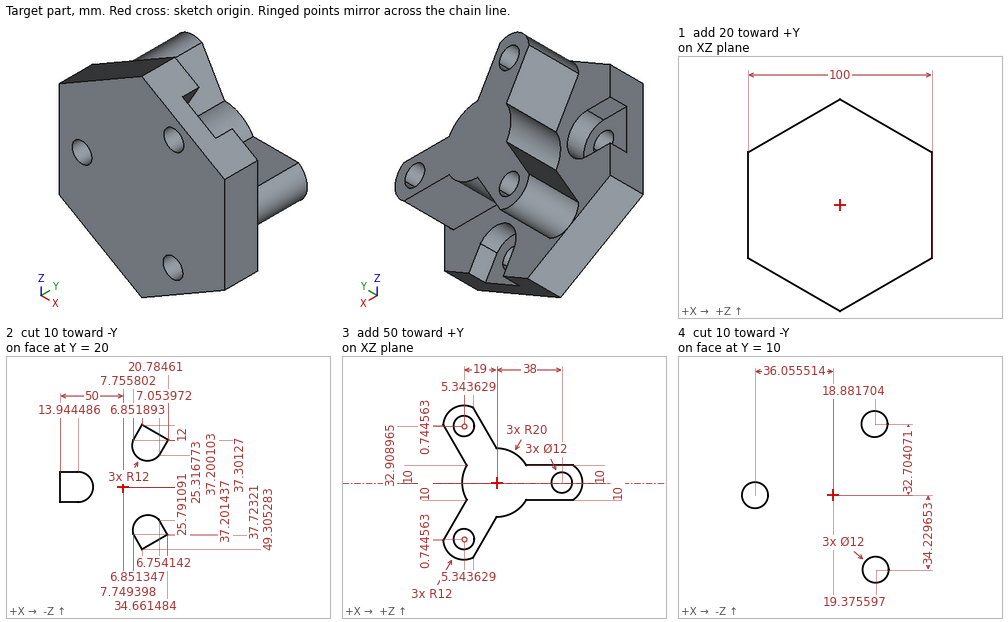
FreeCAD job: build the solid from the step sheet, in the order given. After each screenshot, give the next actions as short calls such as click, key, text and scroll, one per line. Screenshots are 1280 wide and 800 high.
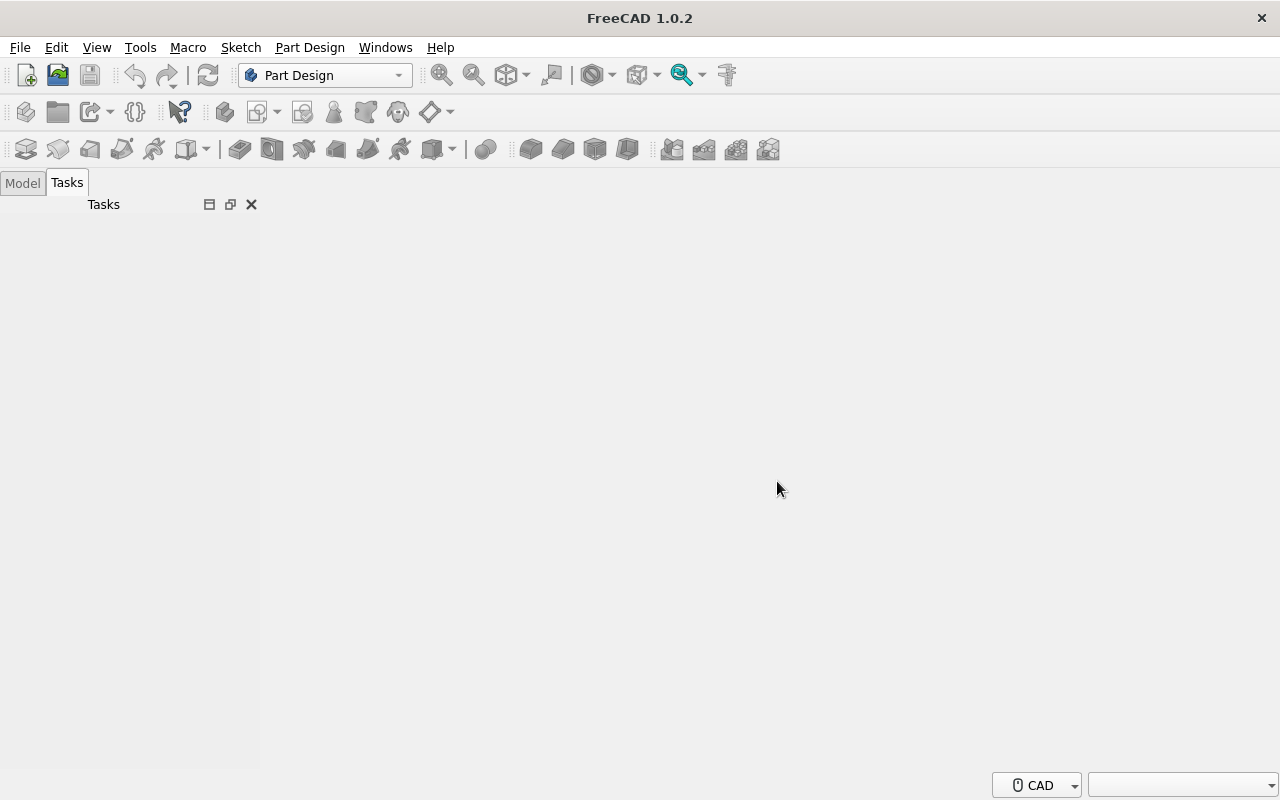
click(26, 76)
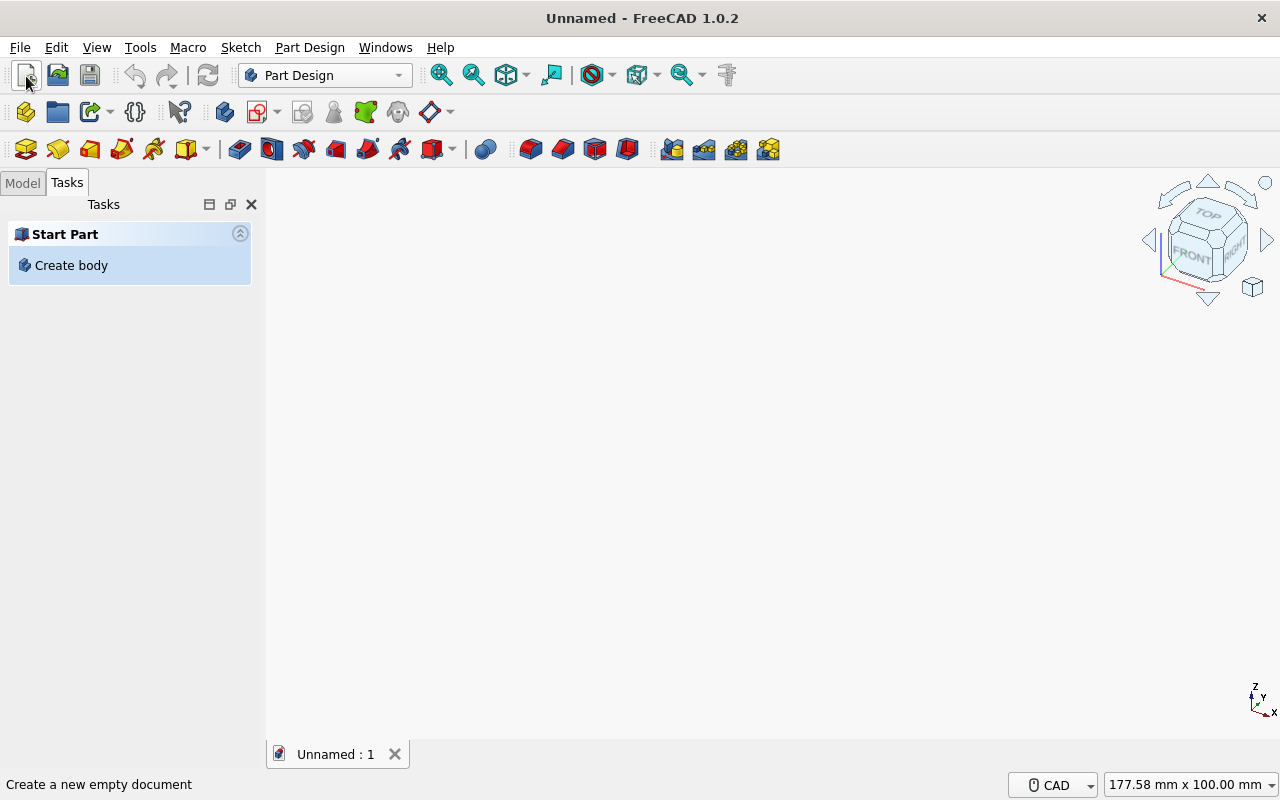
click(258, 112)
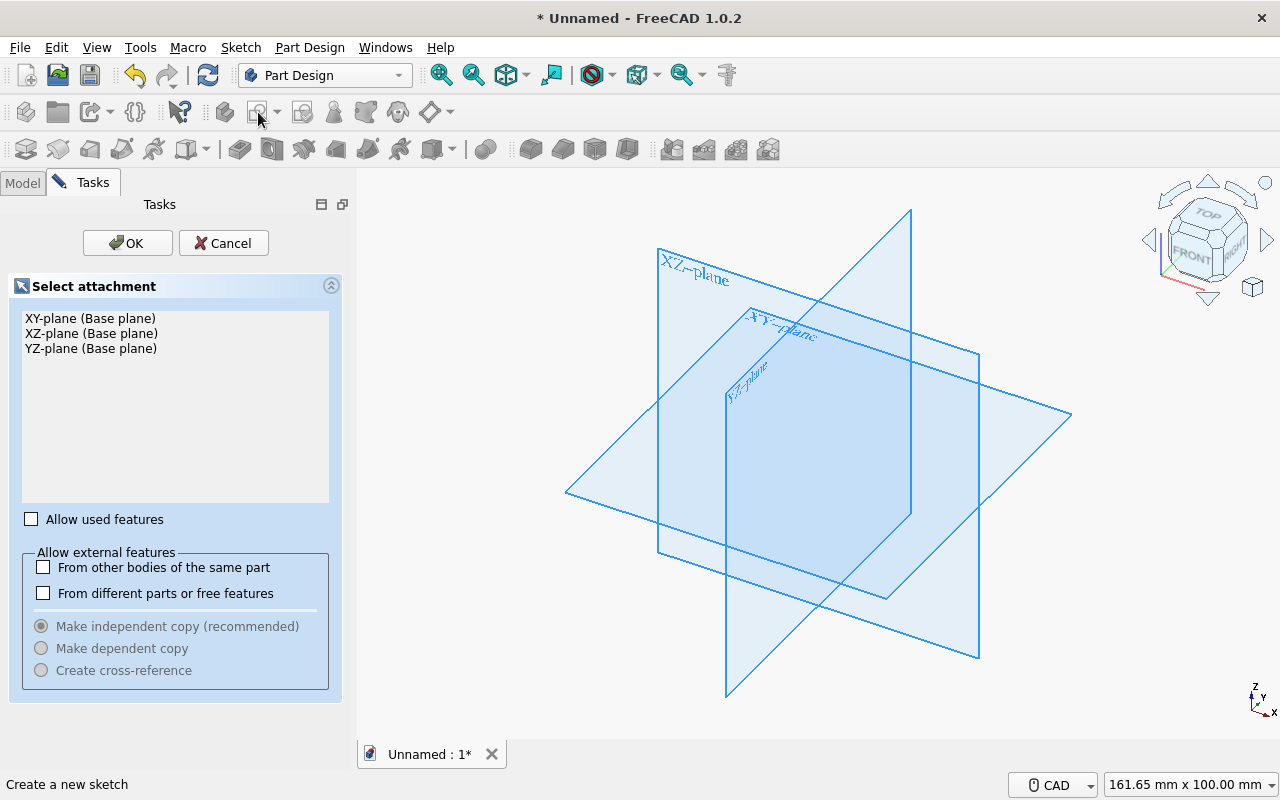
click(82, 334)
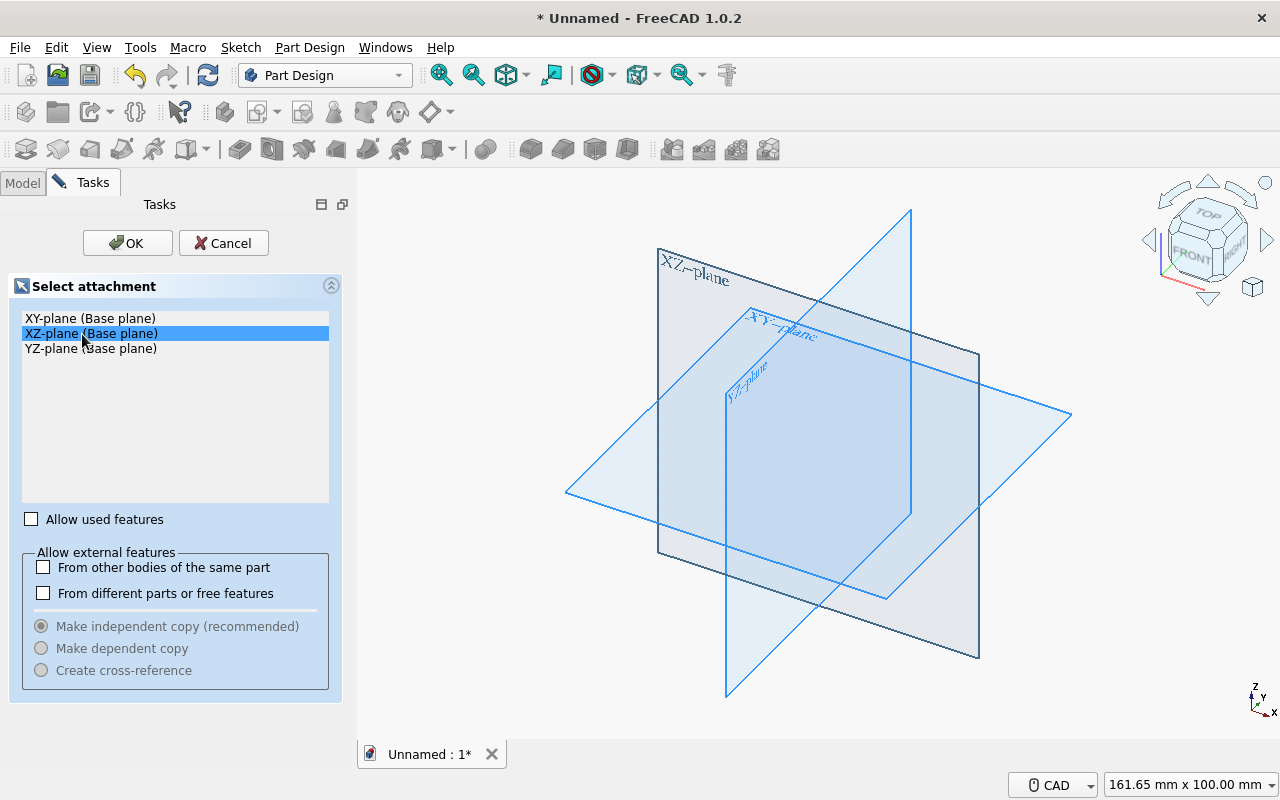
click(128, 243)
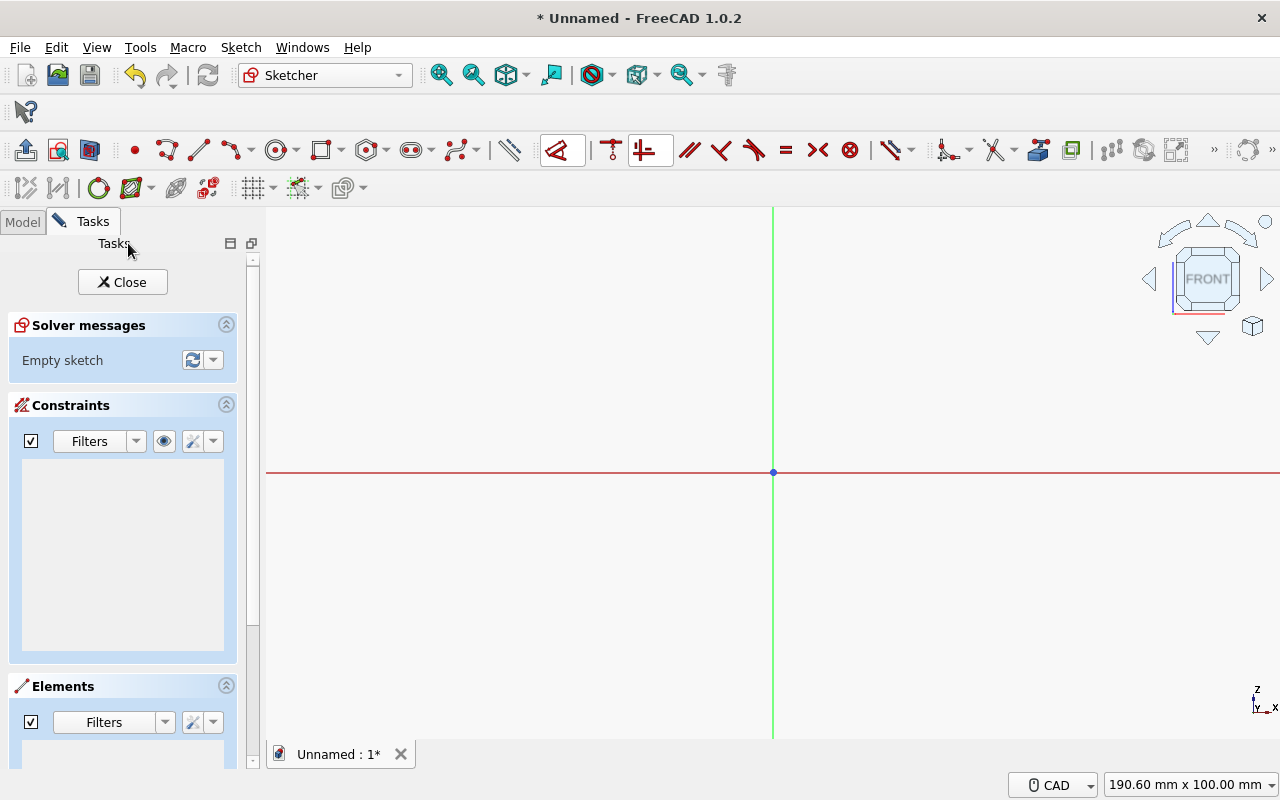
scroll(621, 473, down, 3)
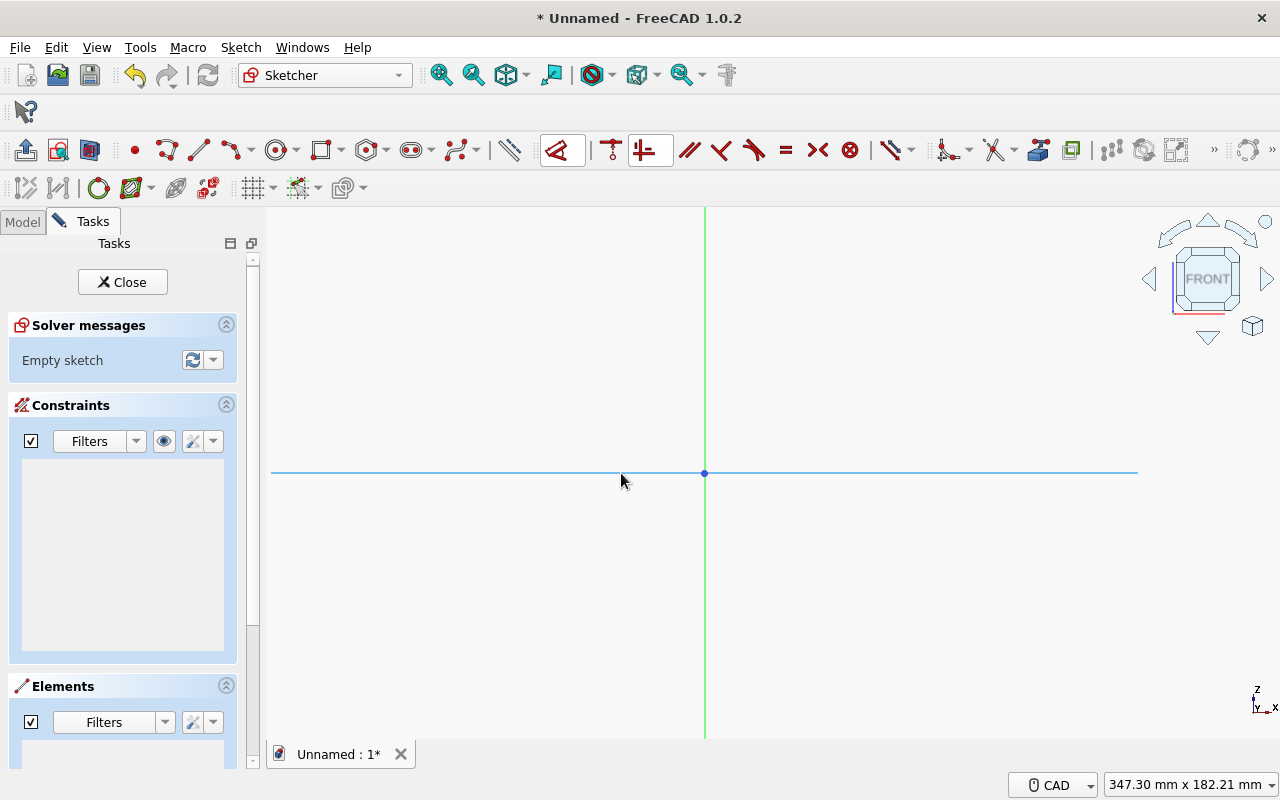
click(366, 150)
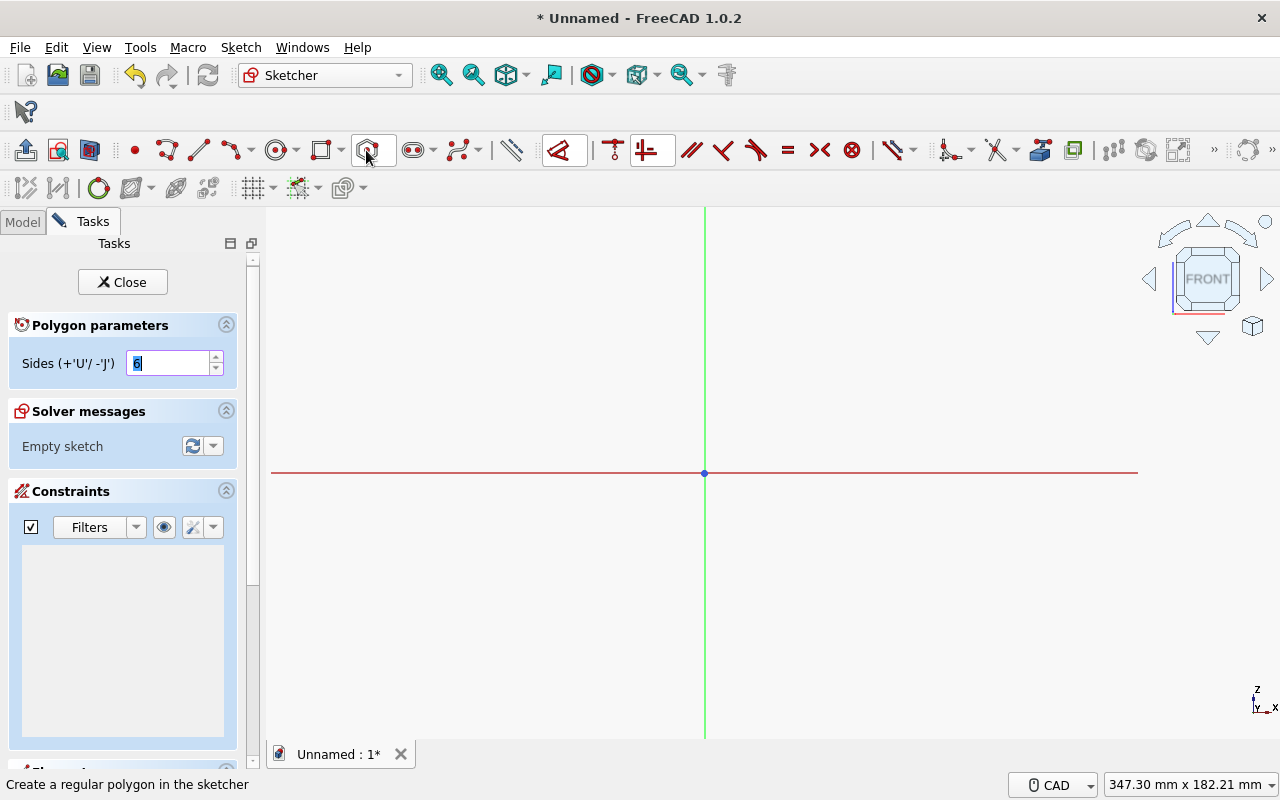
click(705, 473)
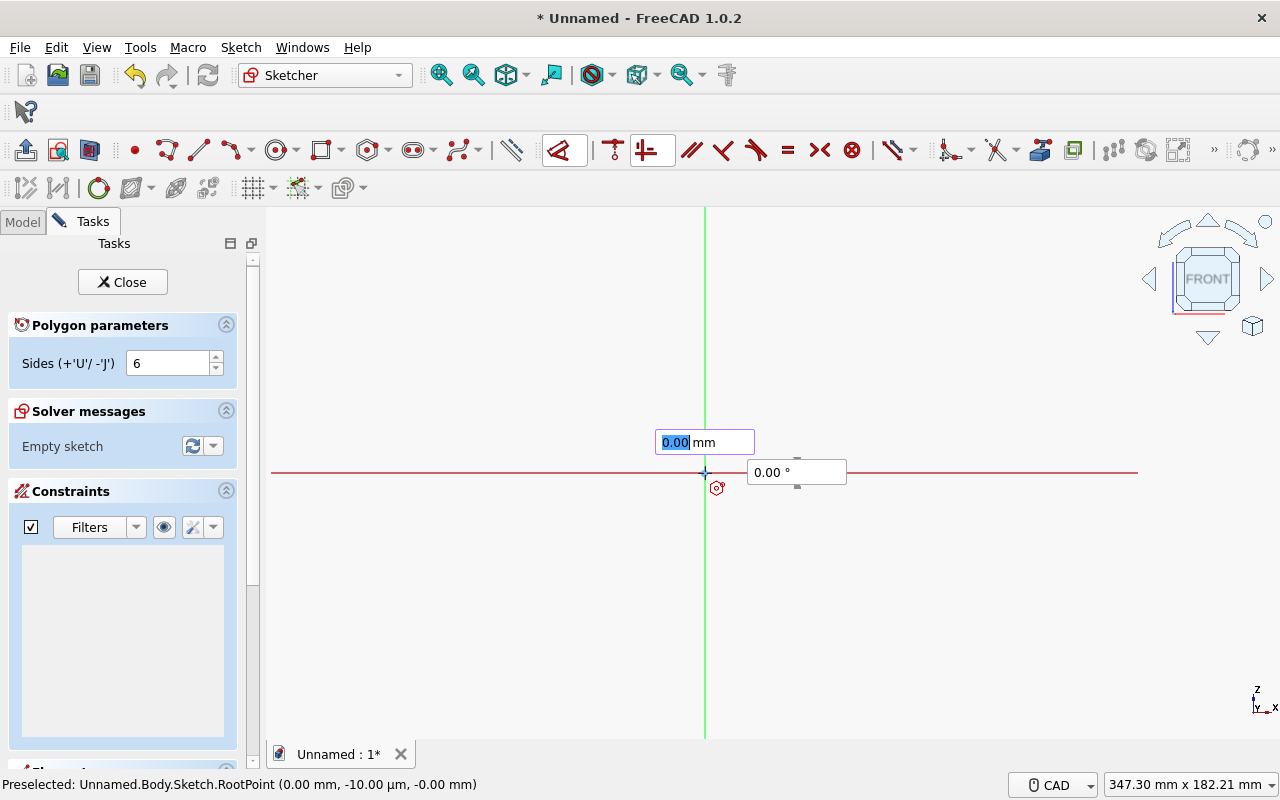
click(705, 642)
key(Escape)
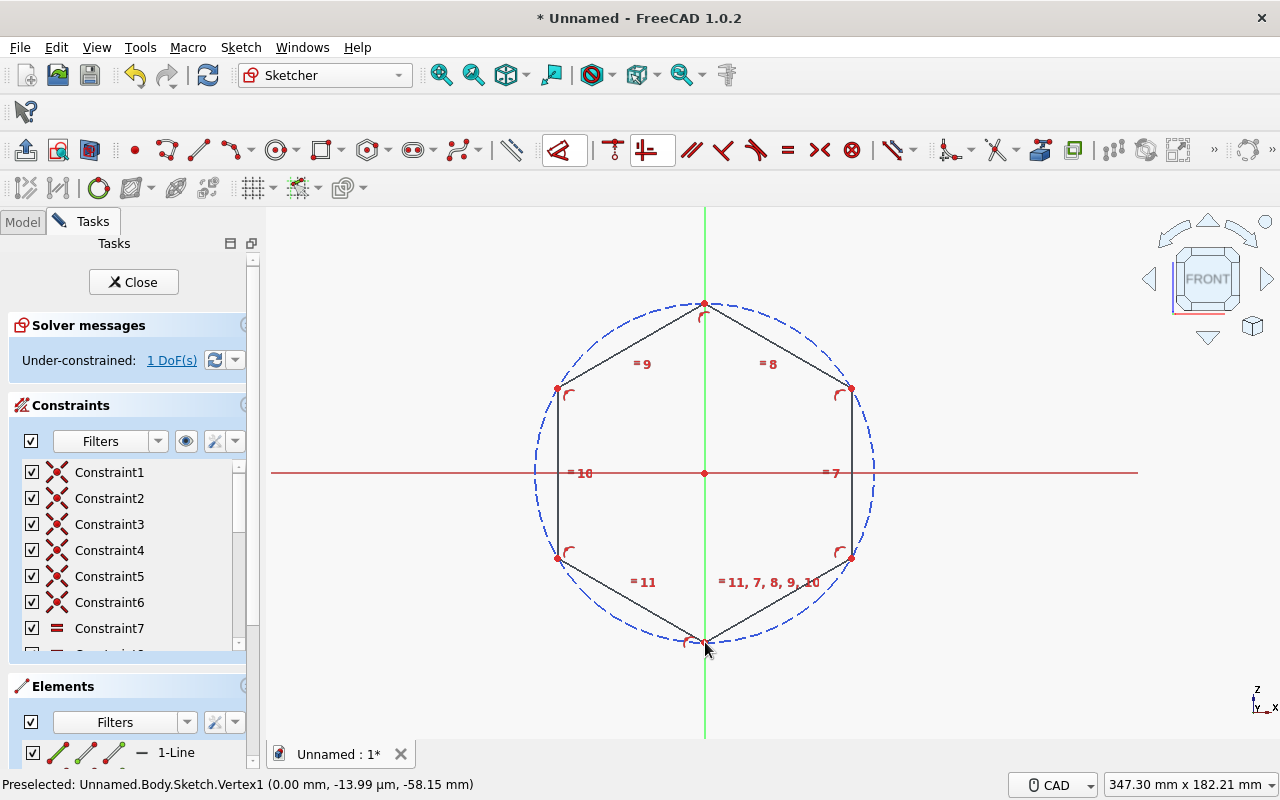
click(558, 150)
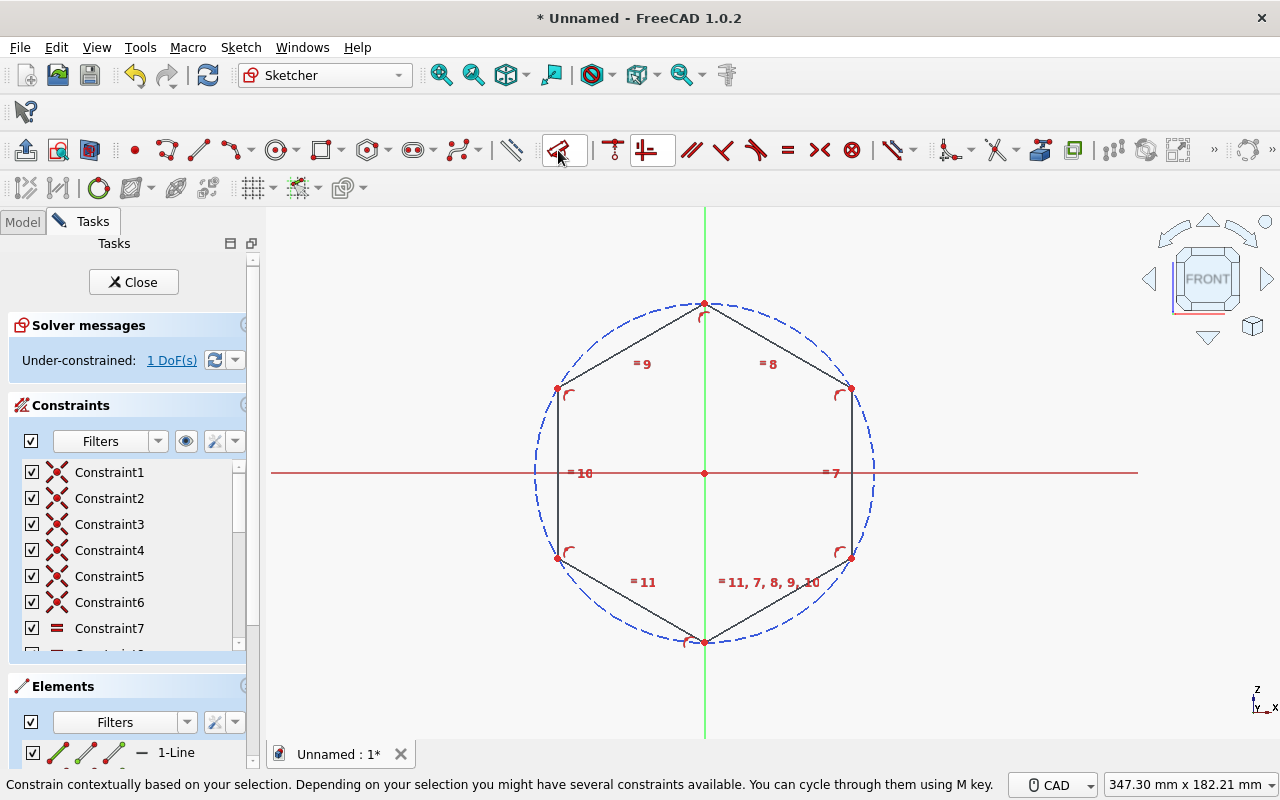
click(558, 388)